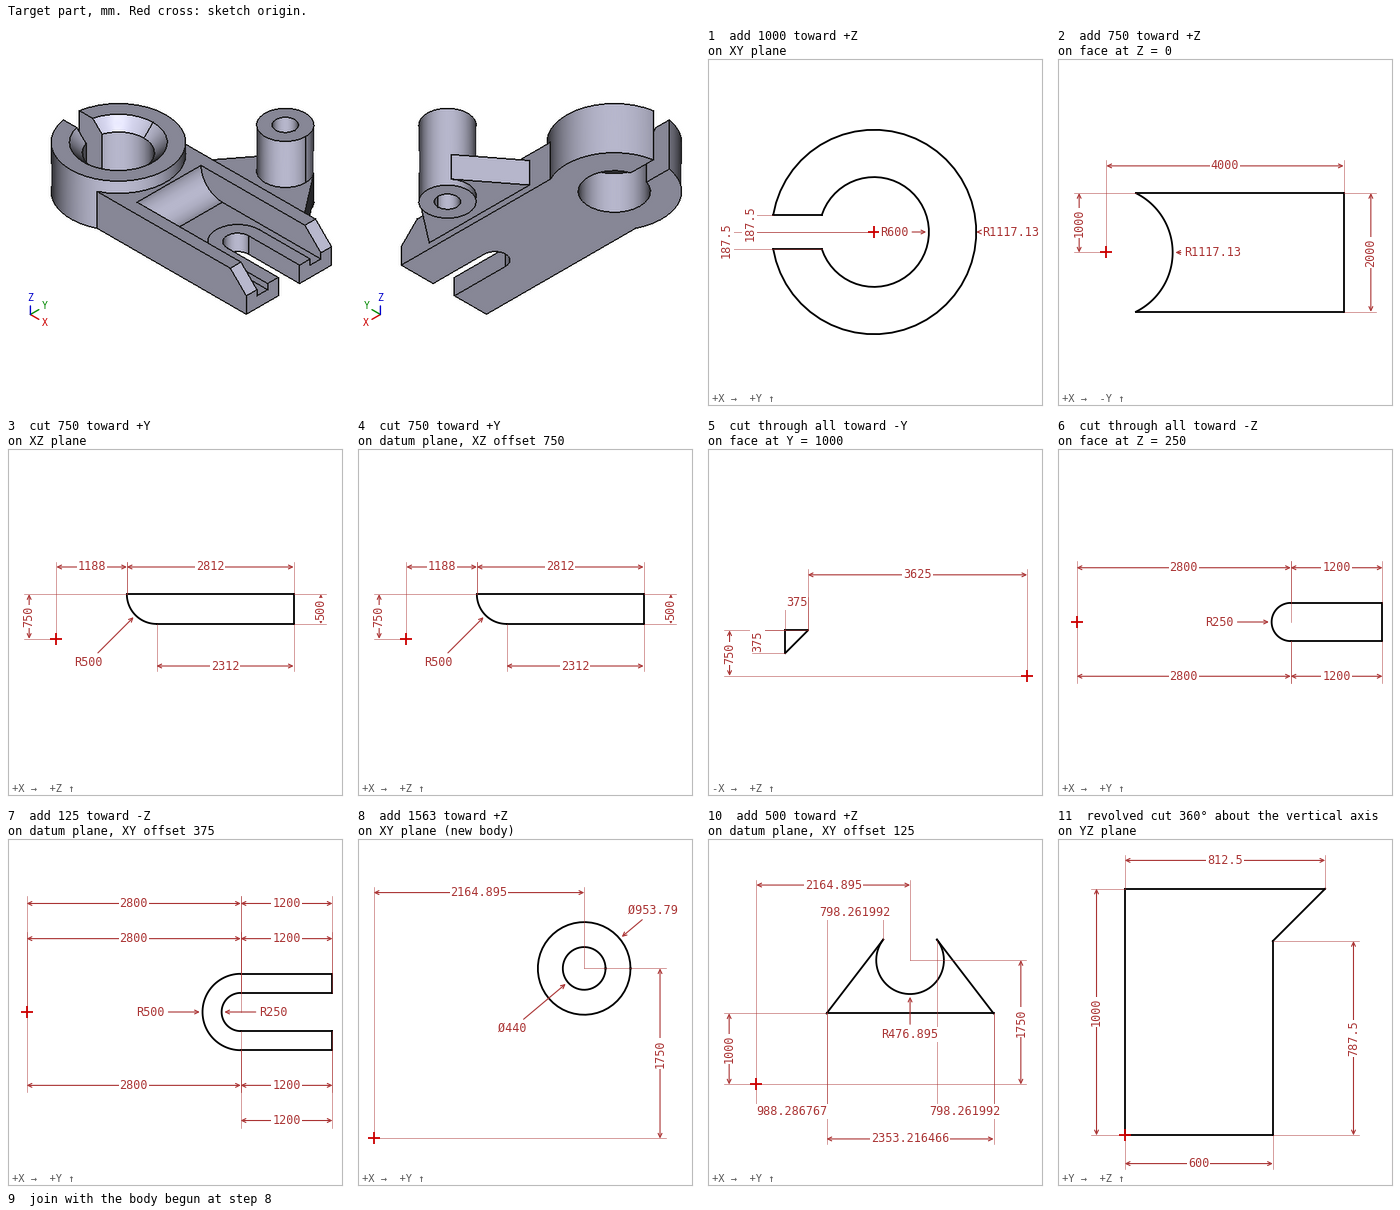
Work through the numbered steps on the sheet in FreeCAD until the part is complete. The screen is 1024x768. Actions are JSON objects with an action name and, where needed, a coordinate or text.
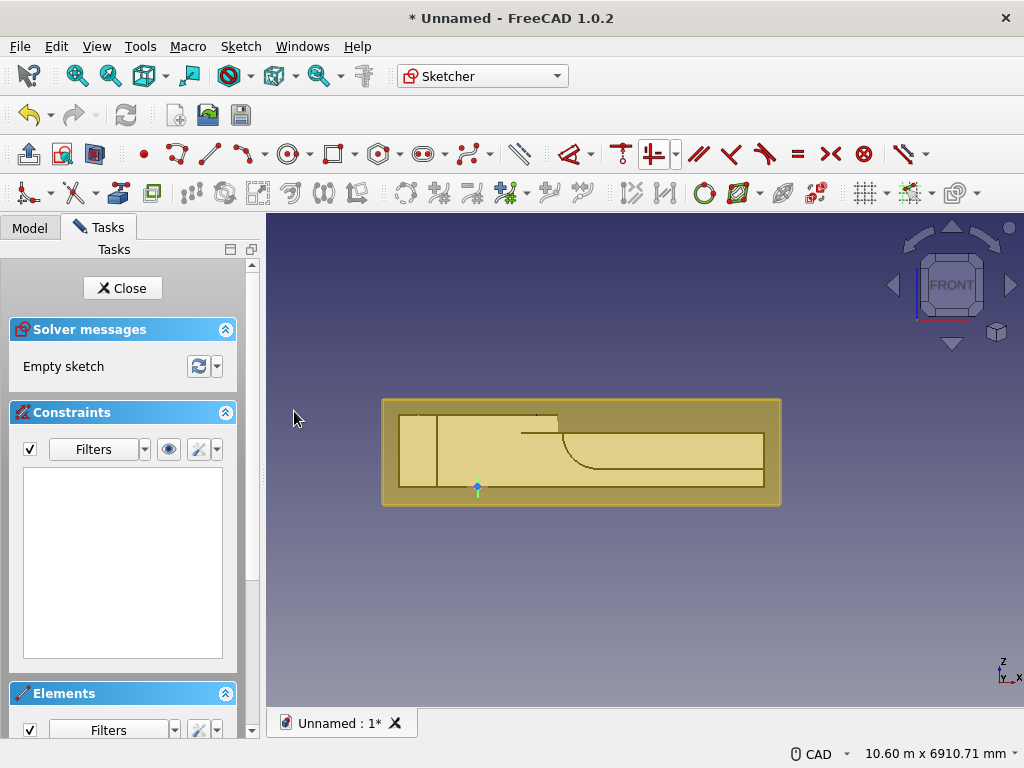
{"action": "scroll", "coordinate": [711, 460], "scroll_direction": "up", "scroll_amount": 2}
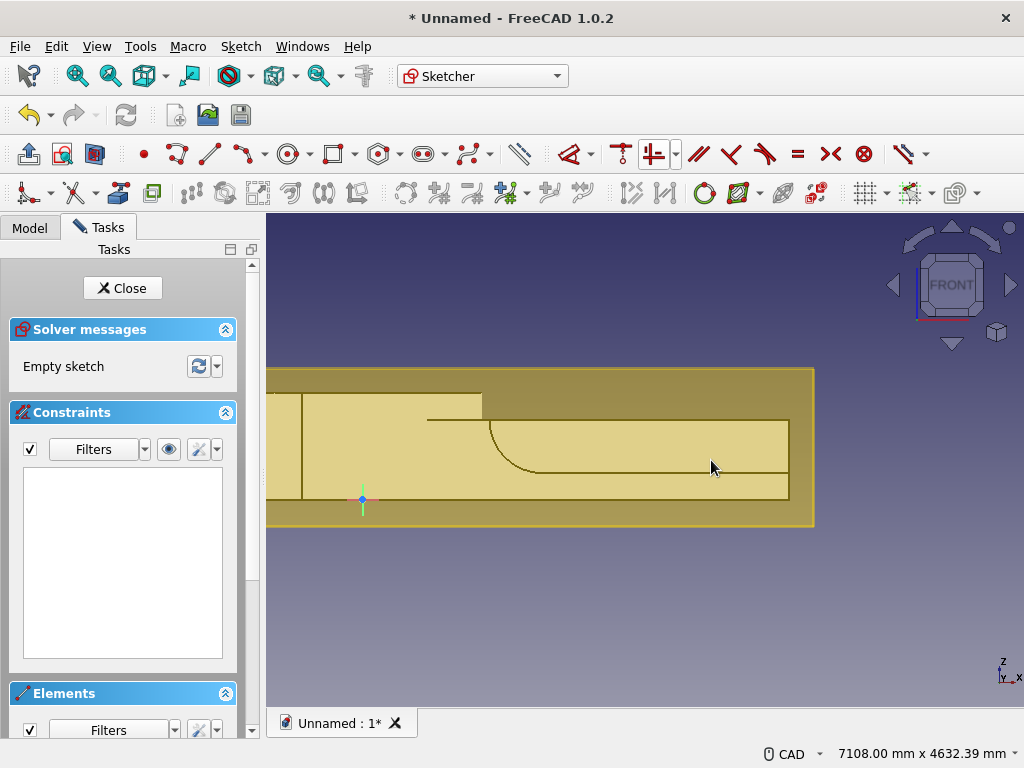
{"action": "key", "text": "g m"}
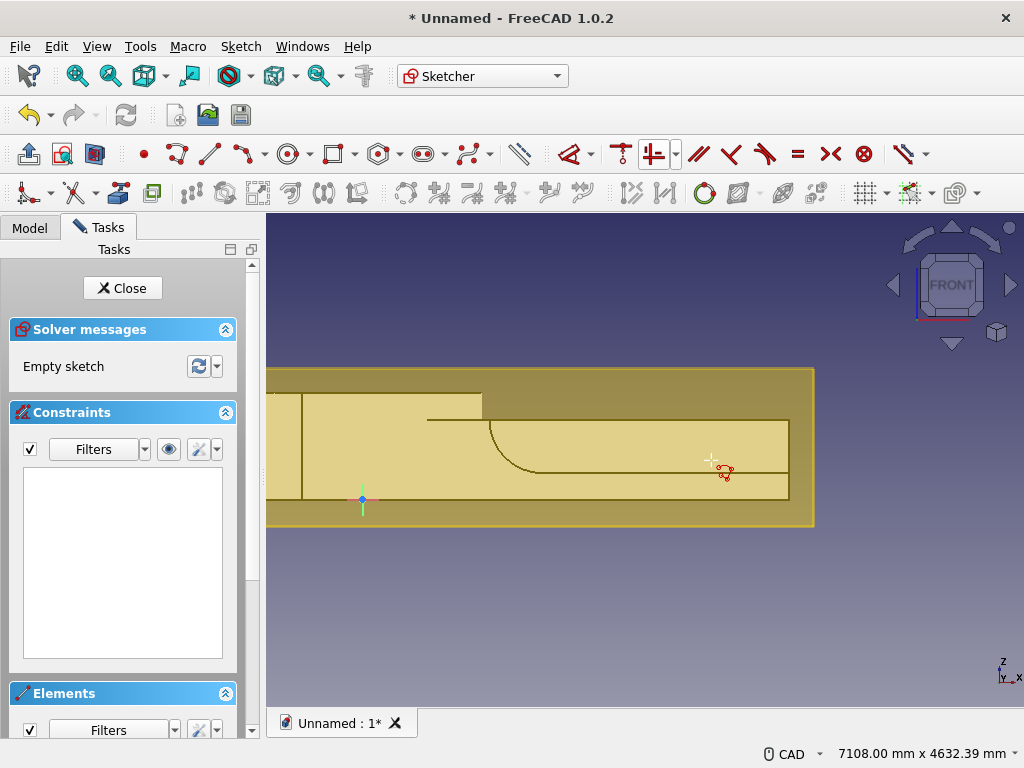
{"action": "left_click", "coordinate": [489, 420]}
{"action": "left_click", "coordinate": [789, 420]}
{"action": "left_click", "coordinate": [789, 473]}
{"action": "left_click", "coordinate": [543, 473]}
{"action": "right_click", "coordinate": [543, 473]}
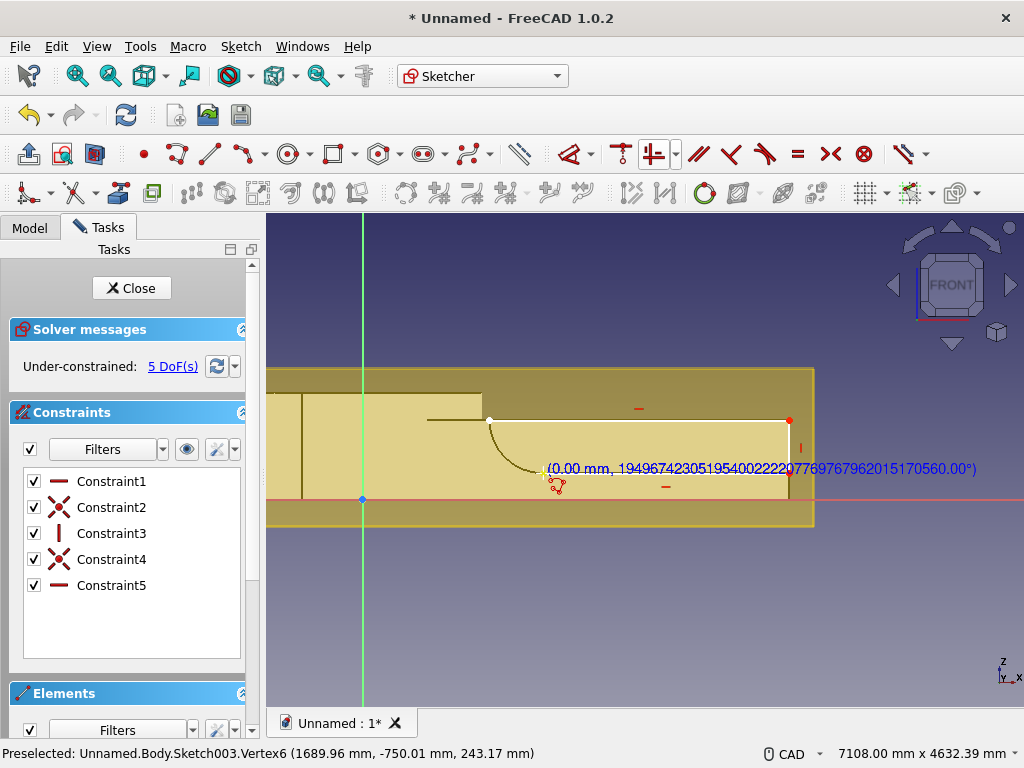
{"action": "key", "text": "g 3 a"}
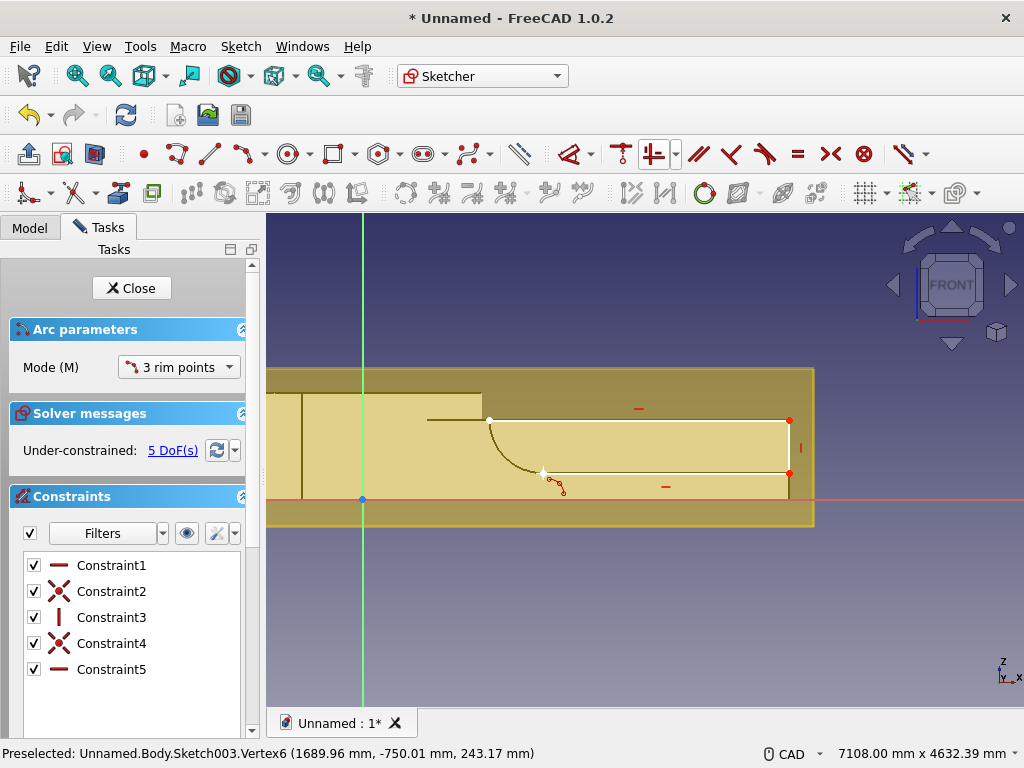
{"action": "left_click", "coordinate": [543, 474]}
{"action": "left_click", "coordinate": [489, 421]}
{"action": "left_click", "coordinate": [505, 458]}
{"action": "key", "text": "Escape"}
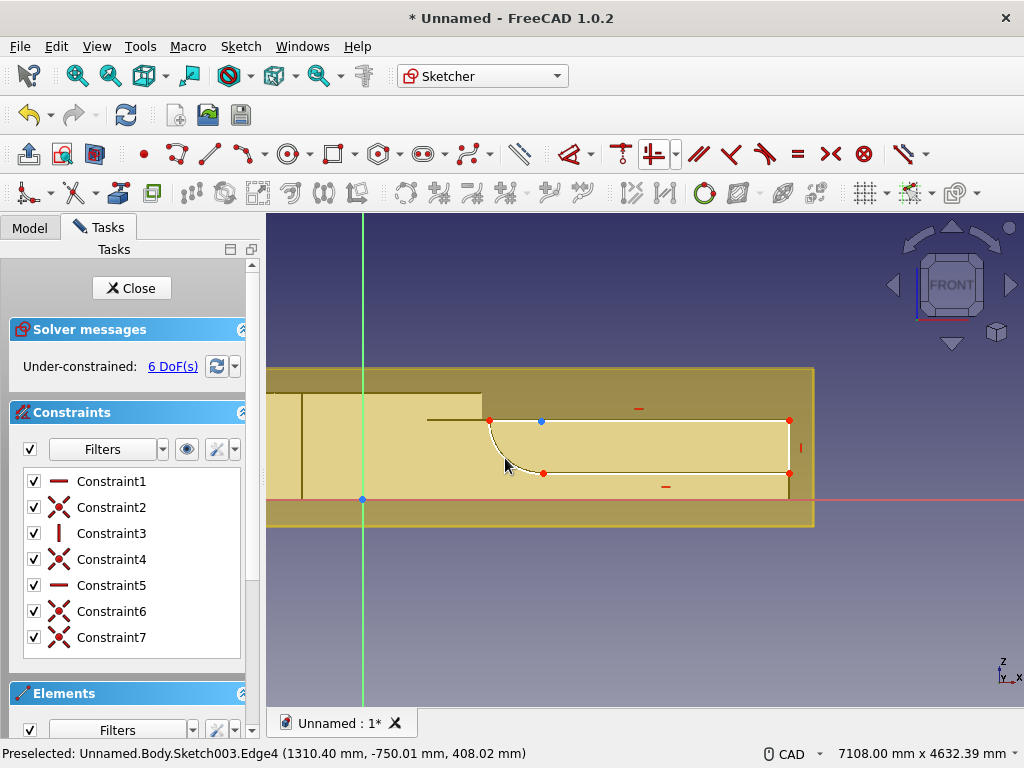
{"action": "key", "text": "d"}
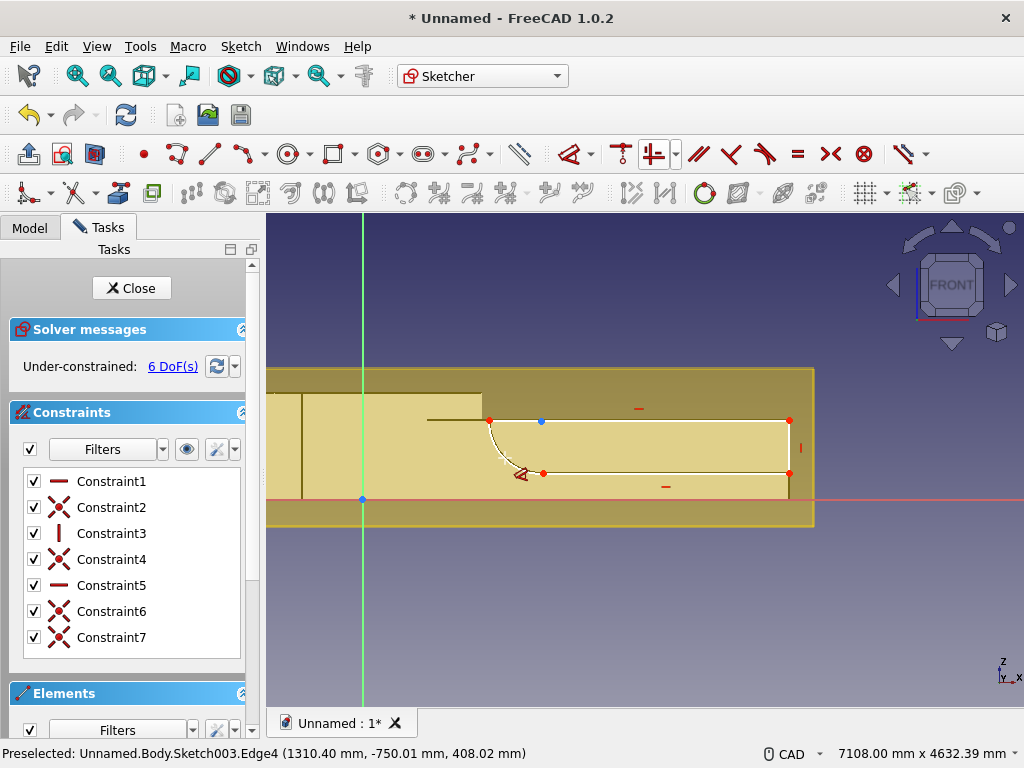
{"action": "left_click", "coordinate": [495, 445]}
{"action": "left_click", "coordinate": [466, 460]}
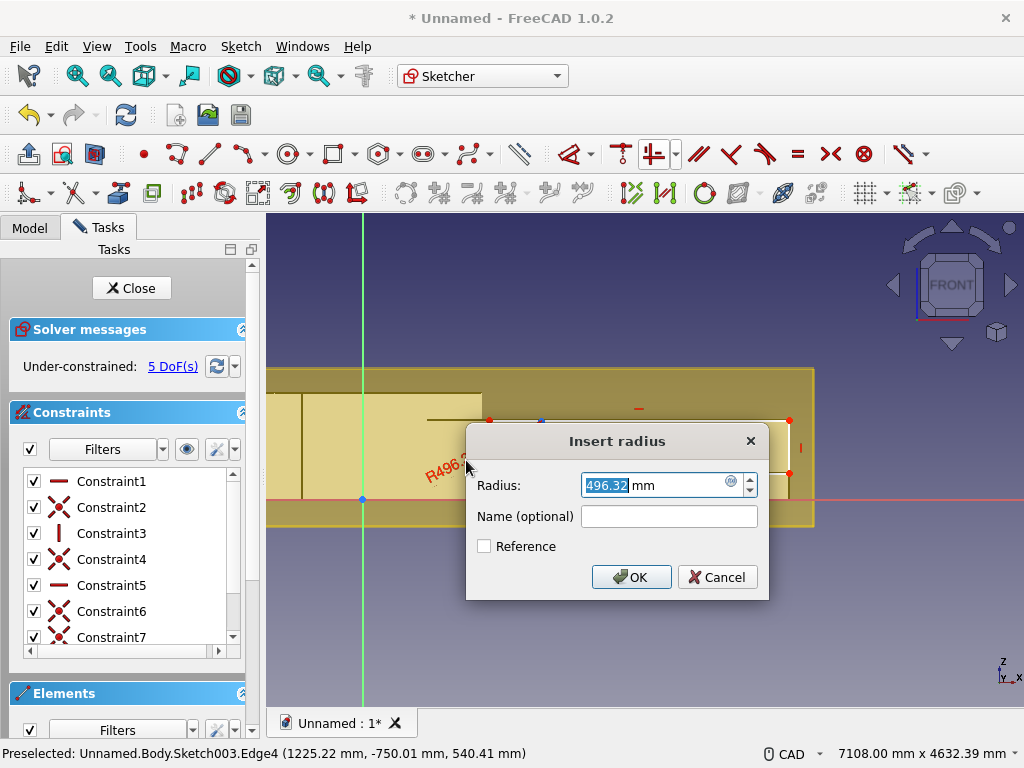
{"action": "type", "text": "500"}
{"action": "key", "text": "Return"}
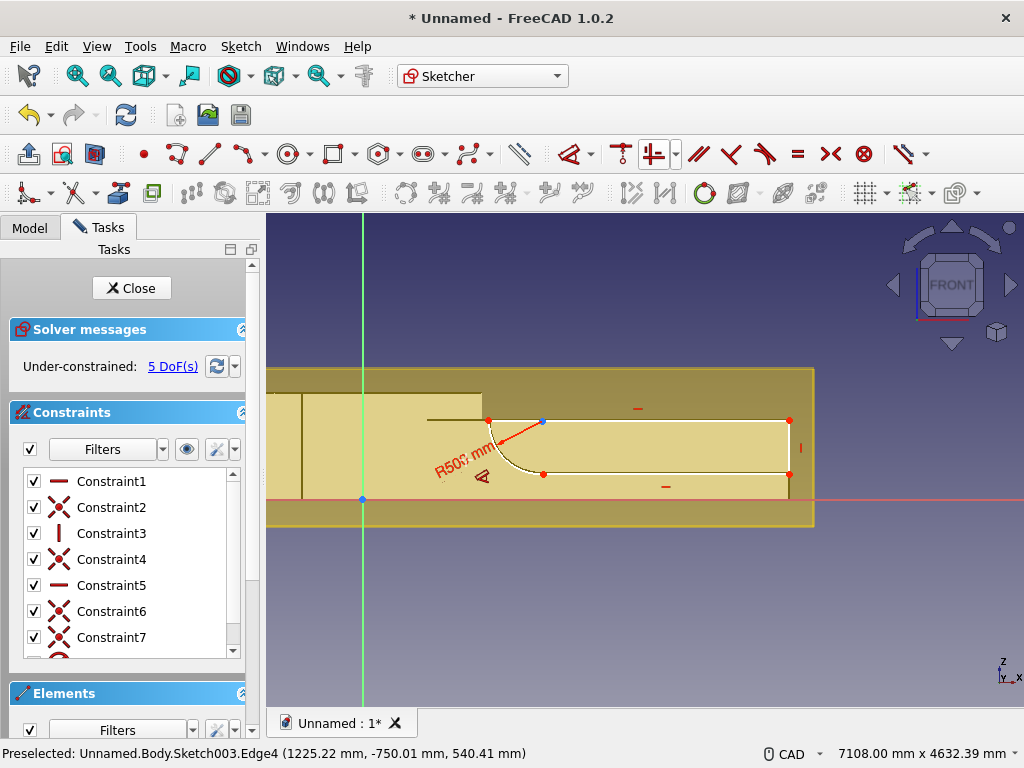
{"action": "left_click", "coordinate": [789, 437]}
{"action": "left_click", "coordinate": [823, 448]}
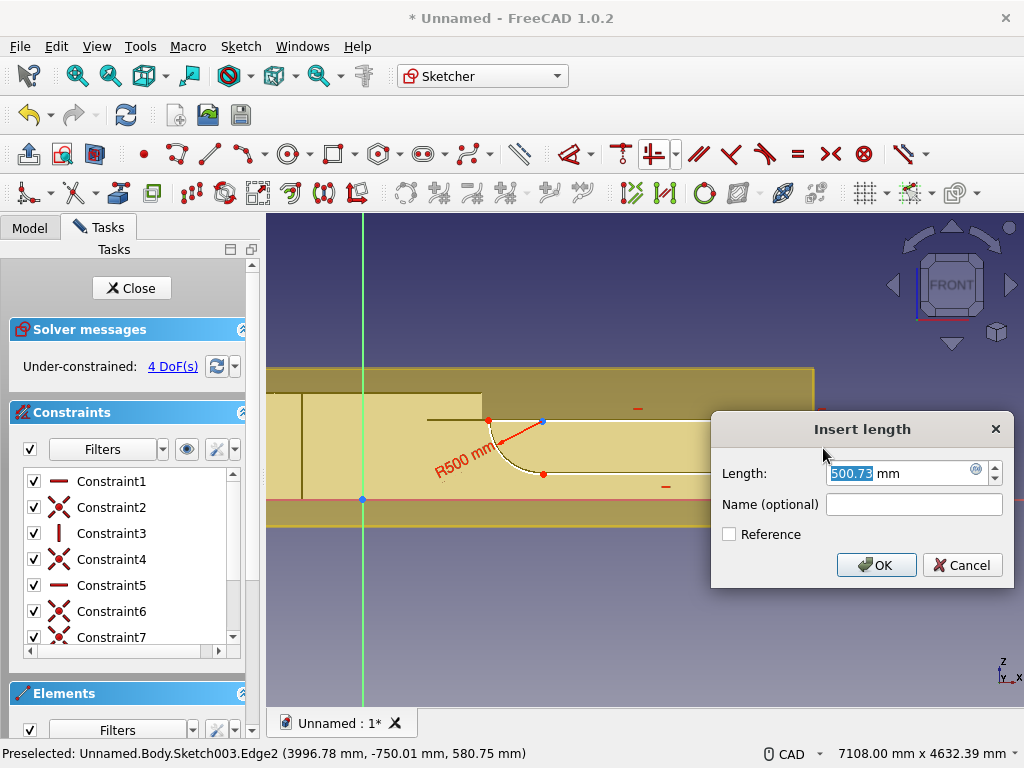
{"action": "type", "text": "500"}
{"action": "key", "text": "Return"}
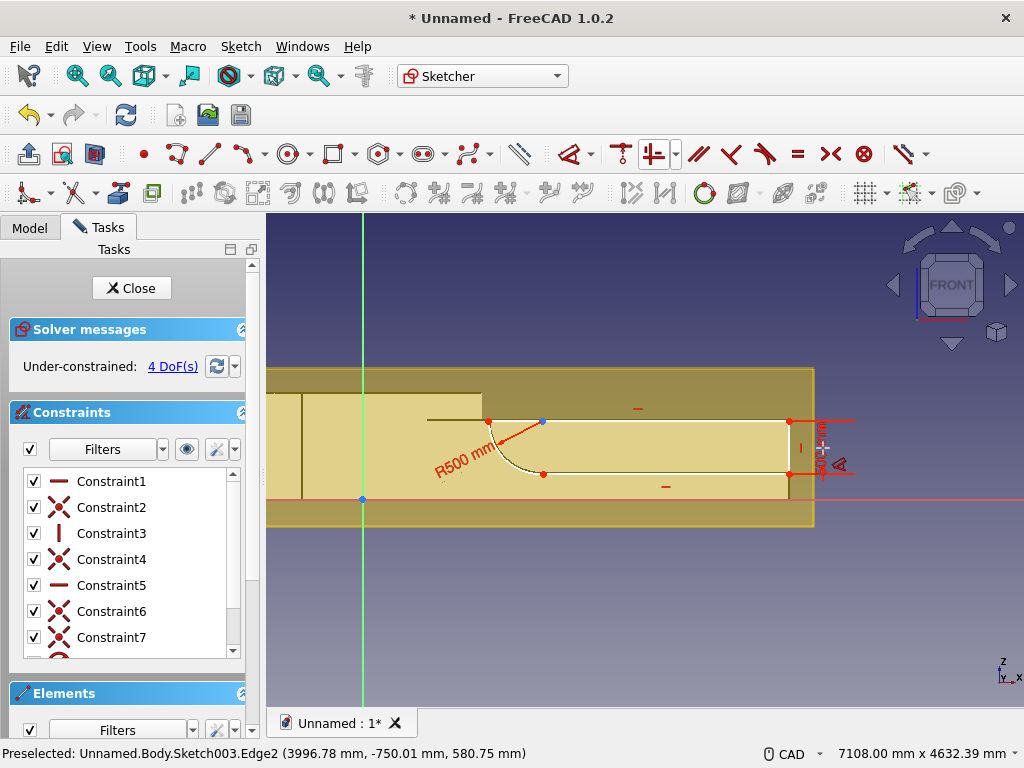
{"action": "left_click", "coordinate": [579, 421]}
{"action": "left_click", "coordinate": [639, 387]}